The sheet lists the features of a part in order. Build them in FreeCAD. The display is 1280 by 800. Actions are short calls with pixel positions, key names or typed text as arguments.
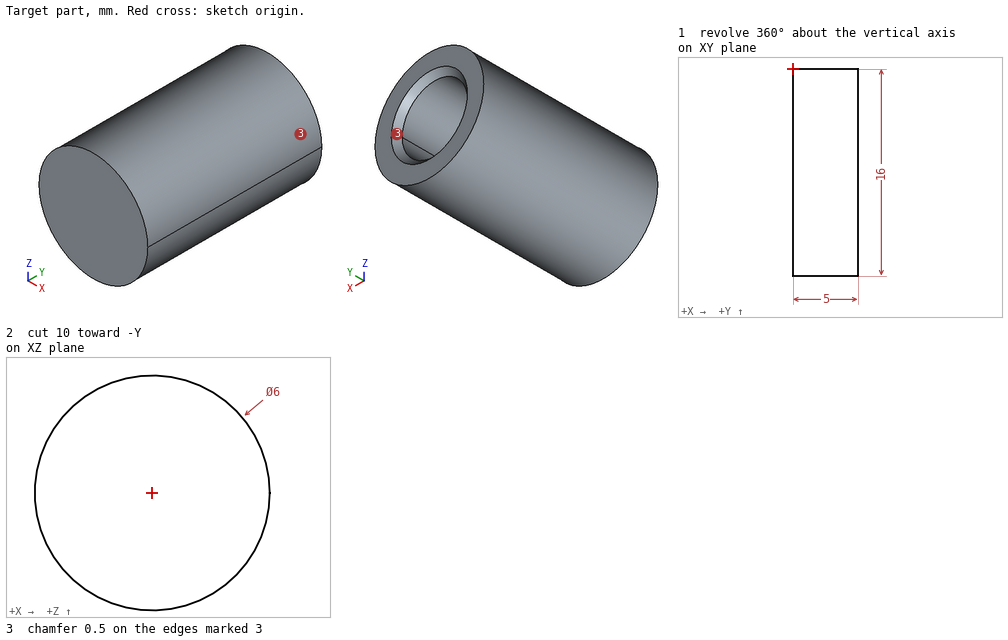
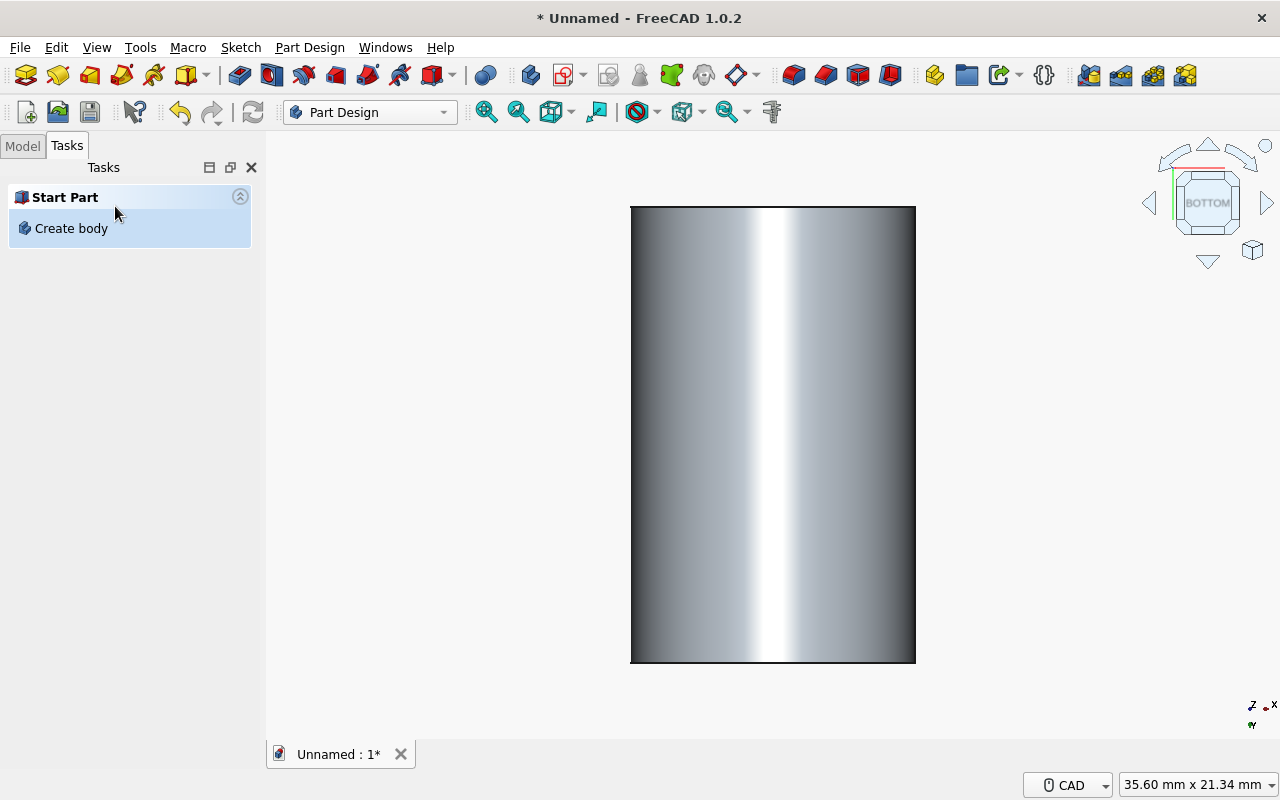
key(4)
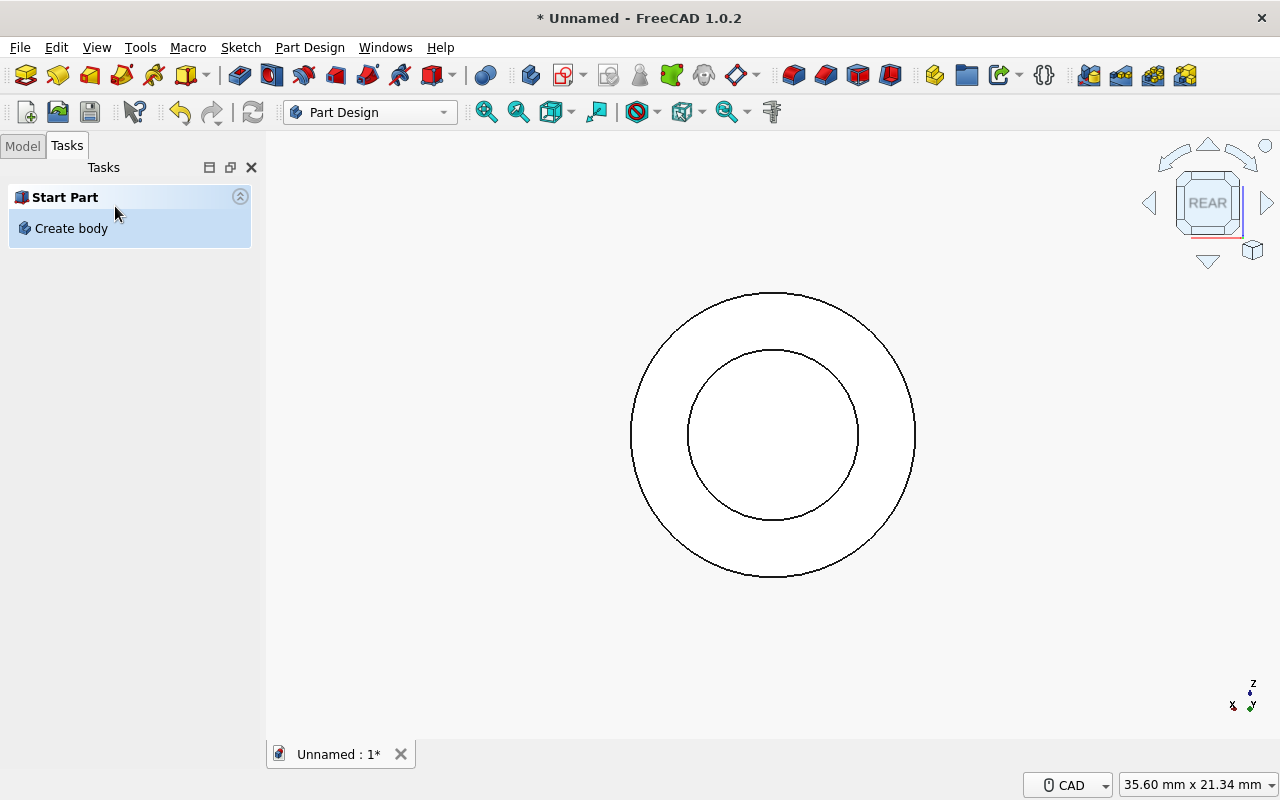
click(858, 434)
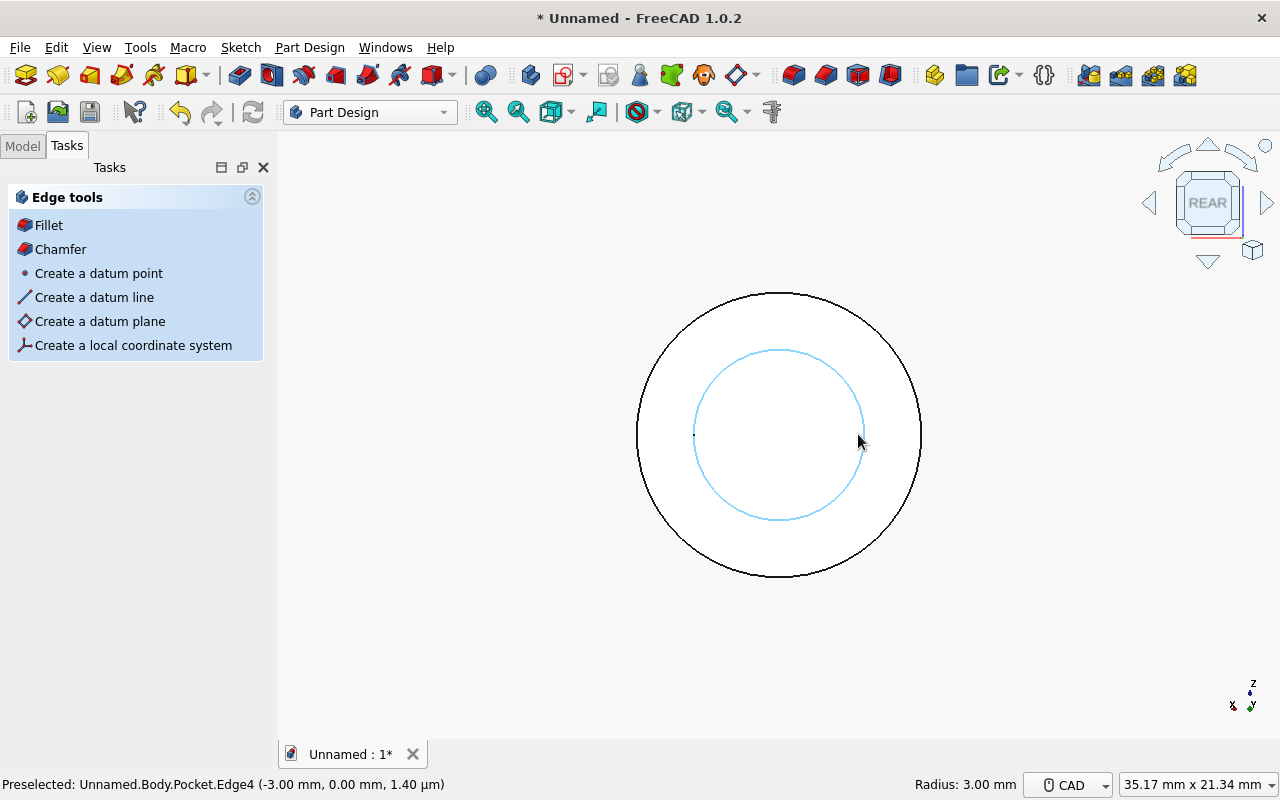
click(826, 76)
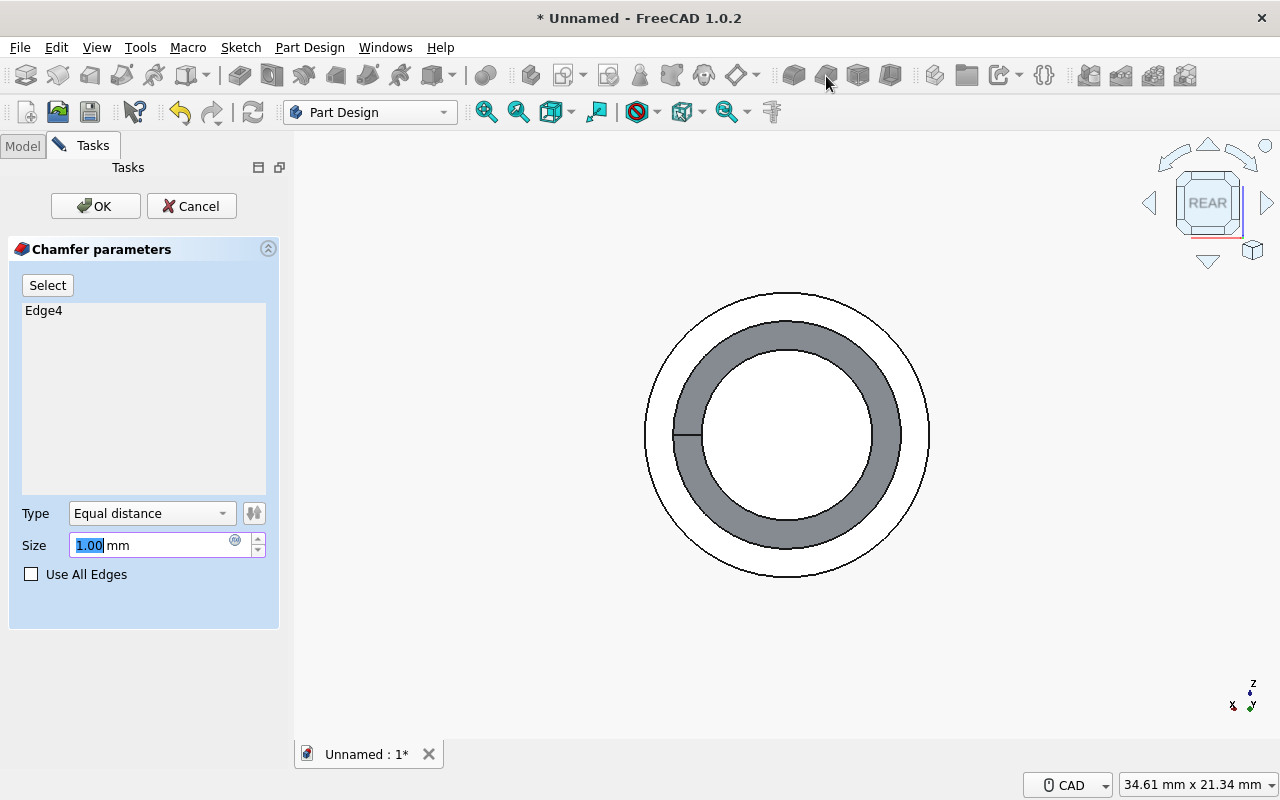
text(0.5)
key(Tab)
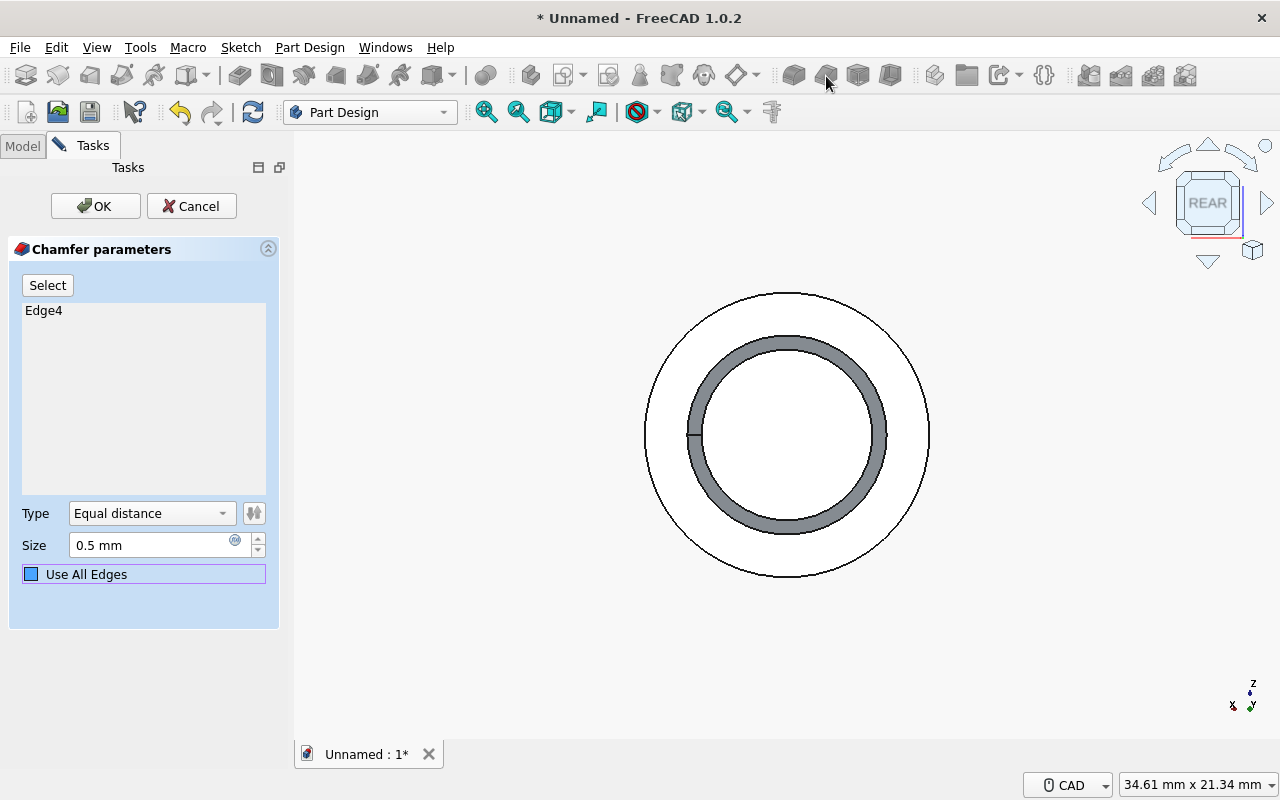
click(96, 206)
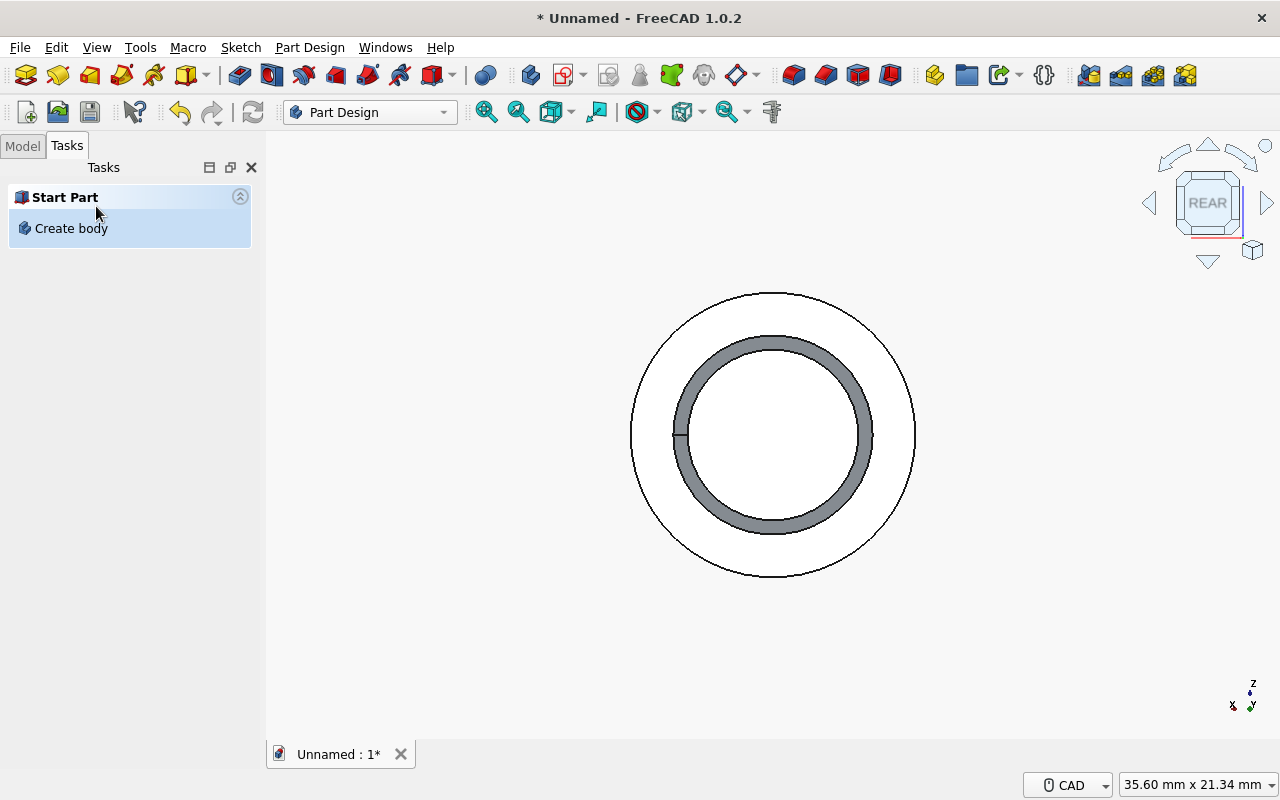
key(0)